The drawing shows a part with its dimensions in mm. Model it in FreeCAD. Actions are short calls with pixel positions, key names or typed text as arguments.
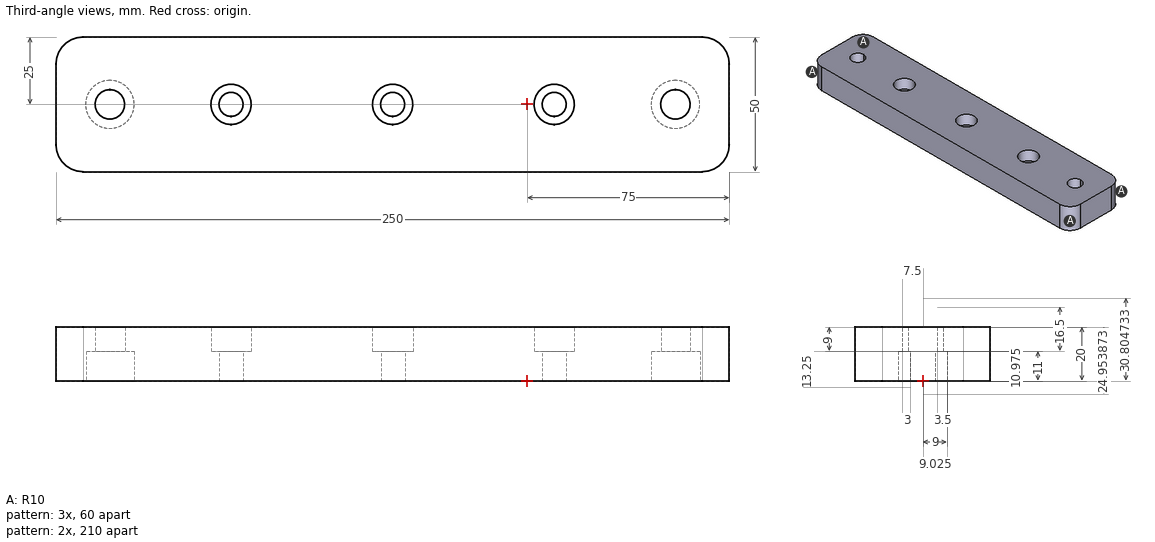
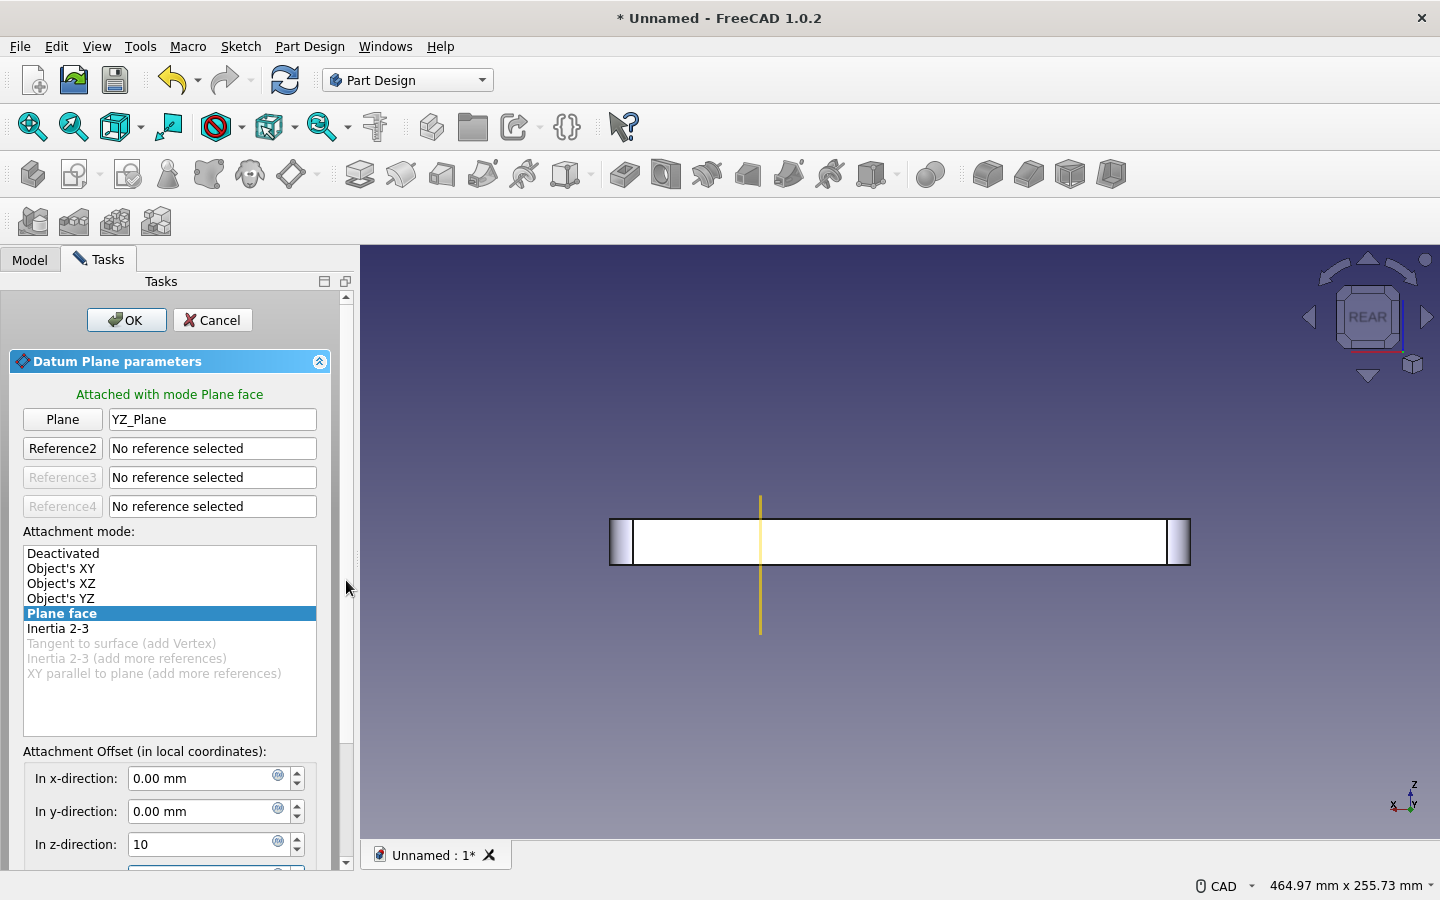
click(127, 320)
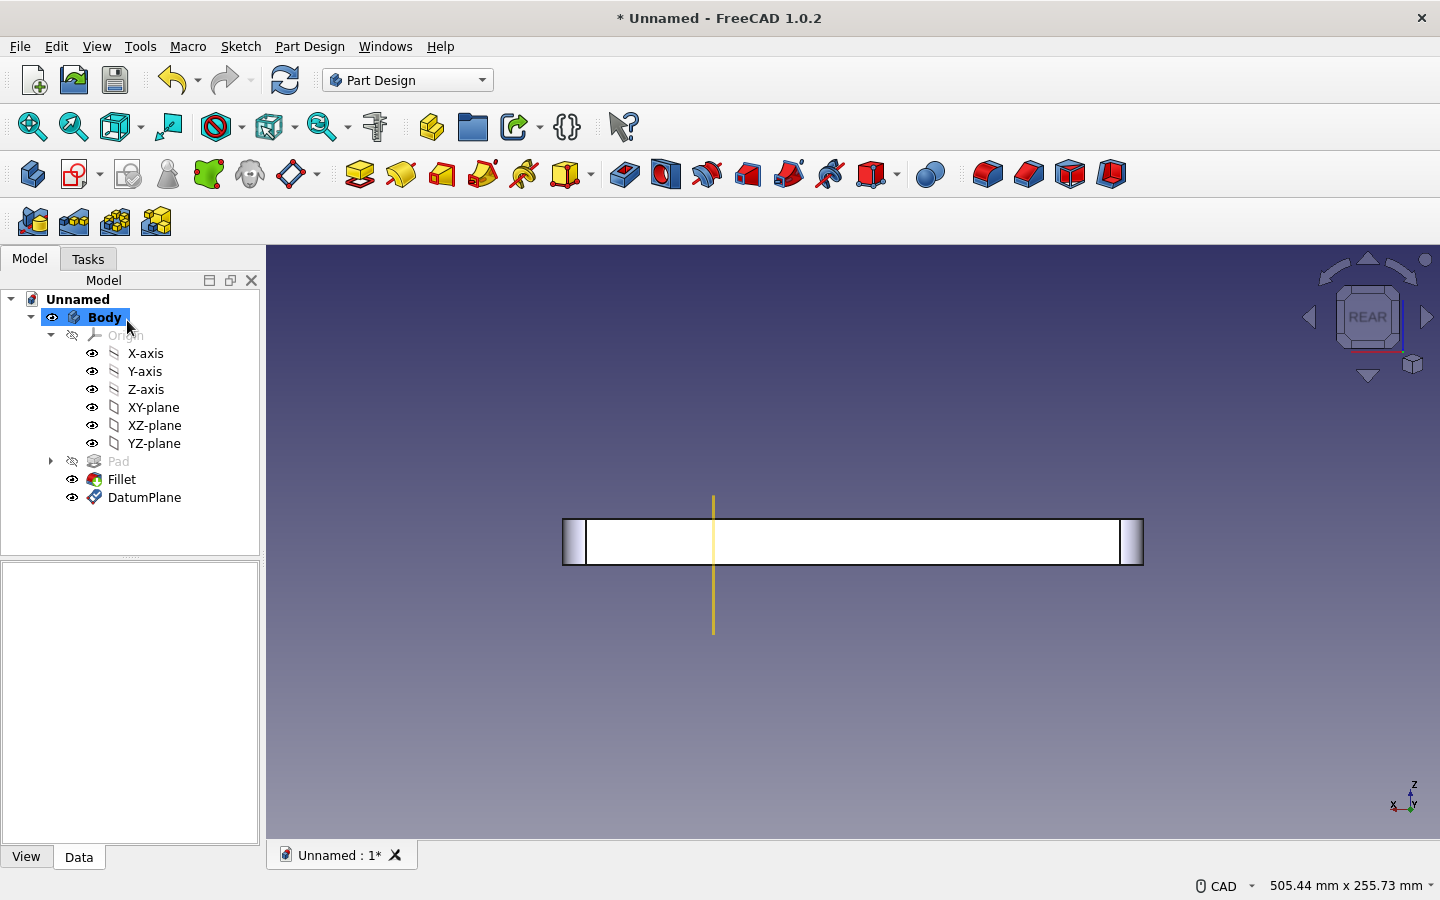
click(117, 497)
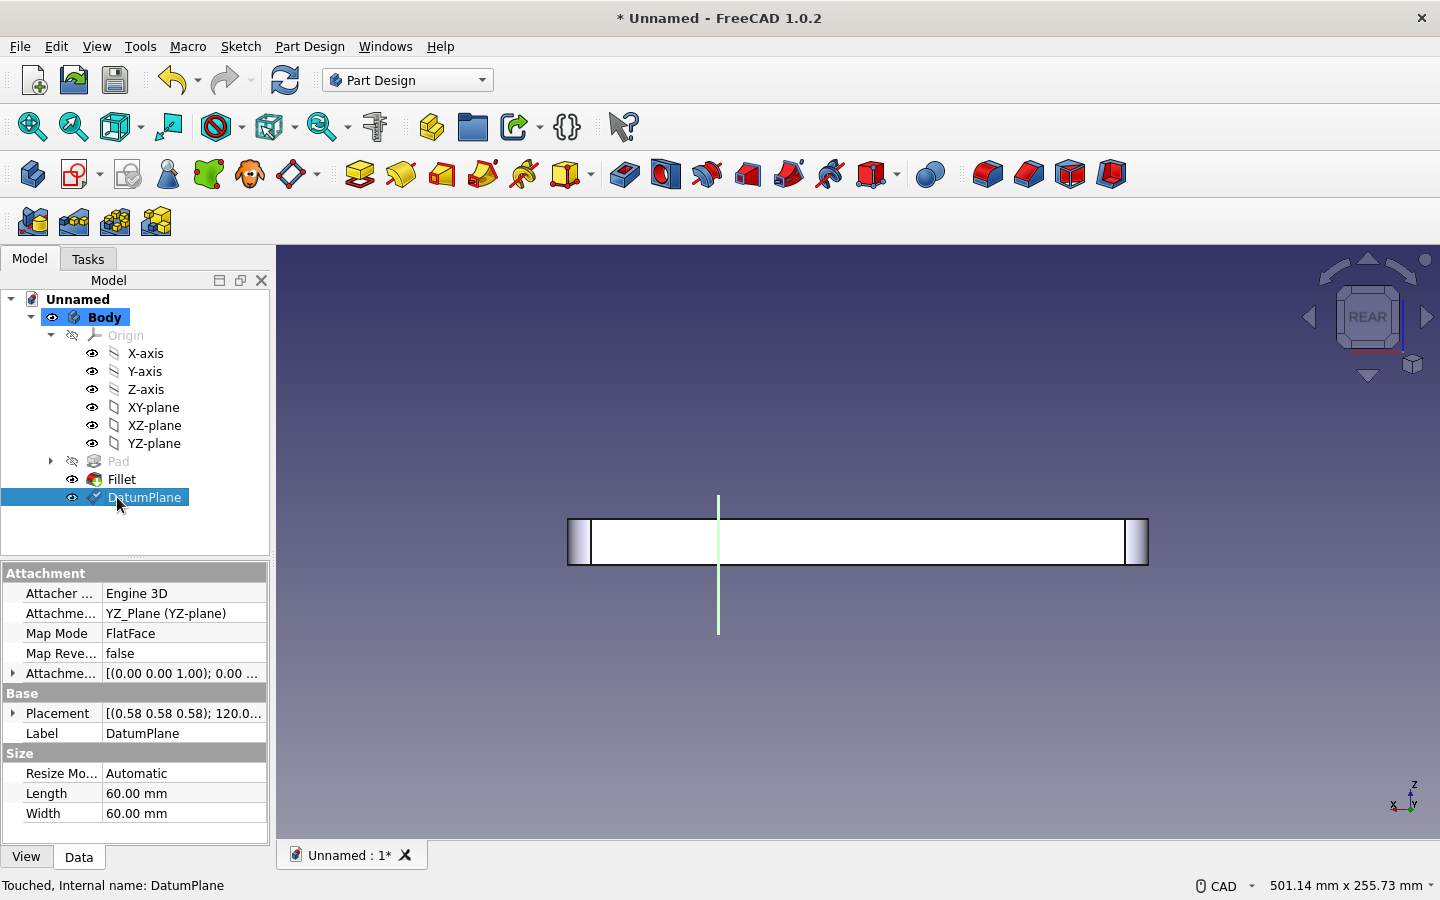
click(74, 174)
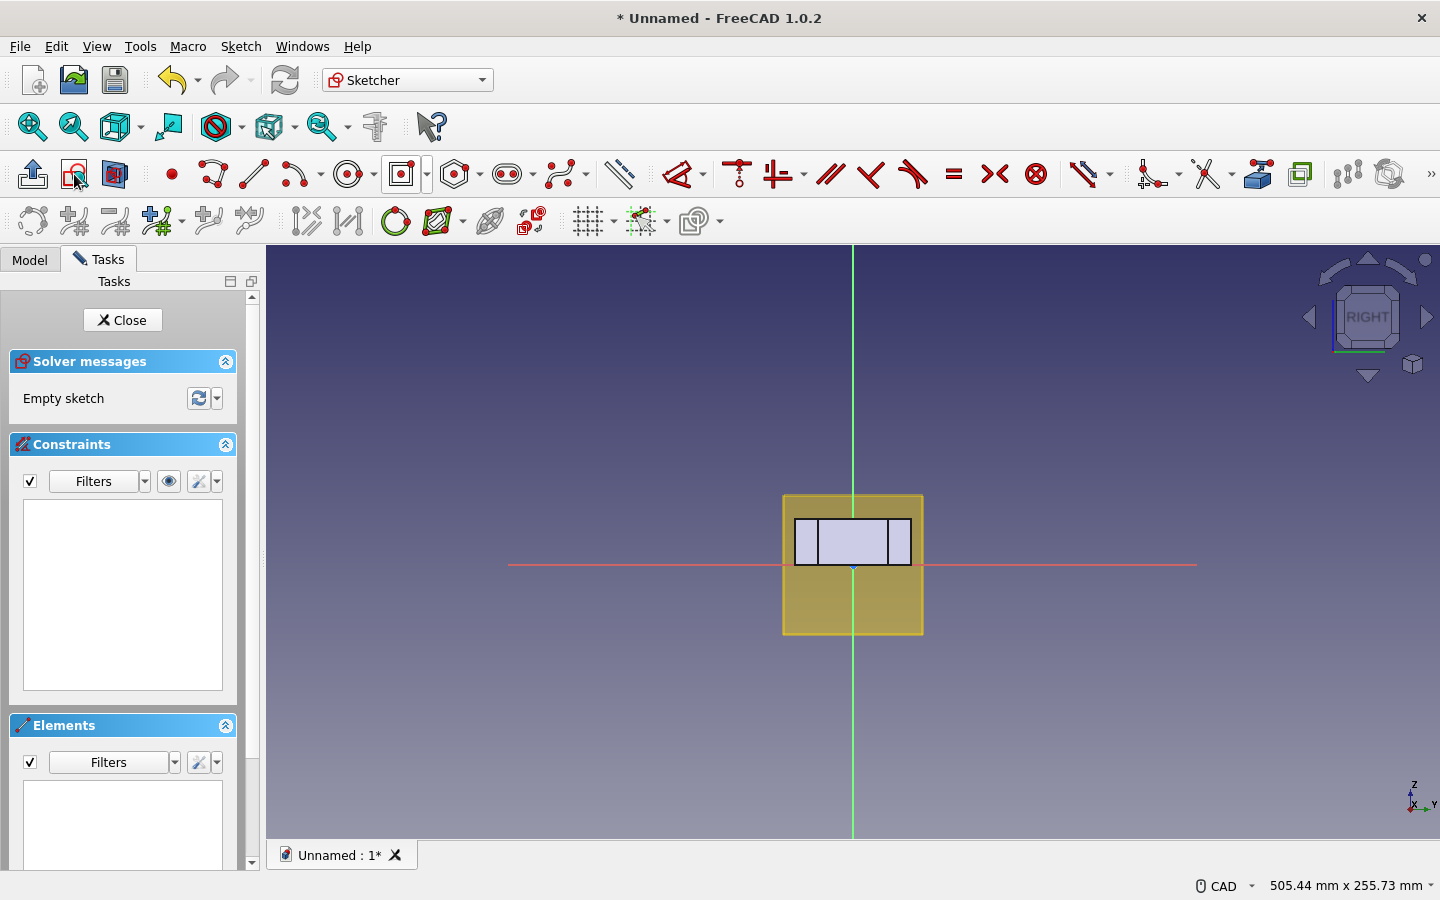
key(q)
key(s)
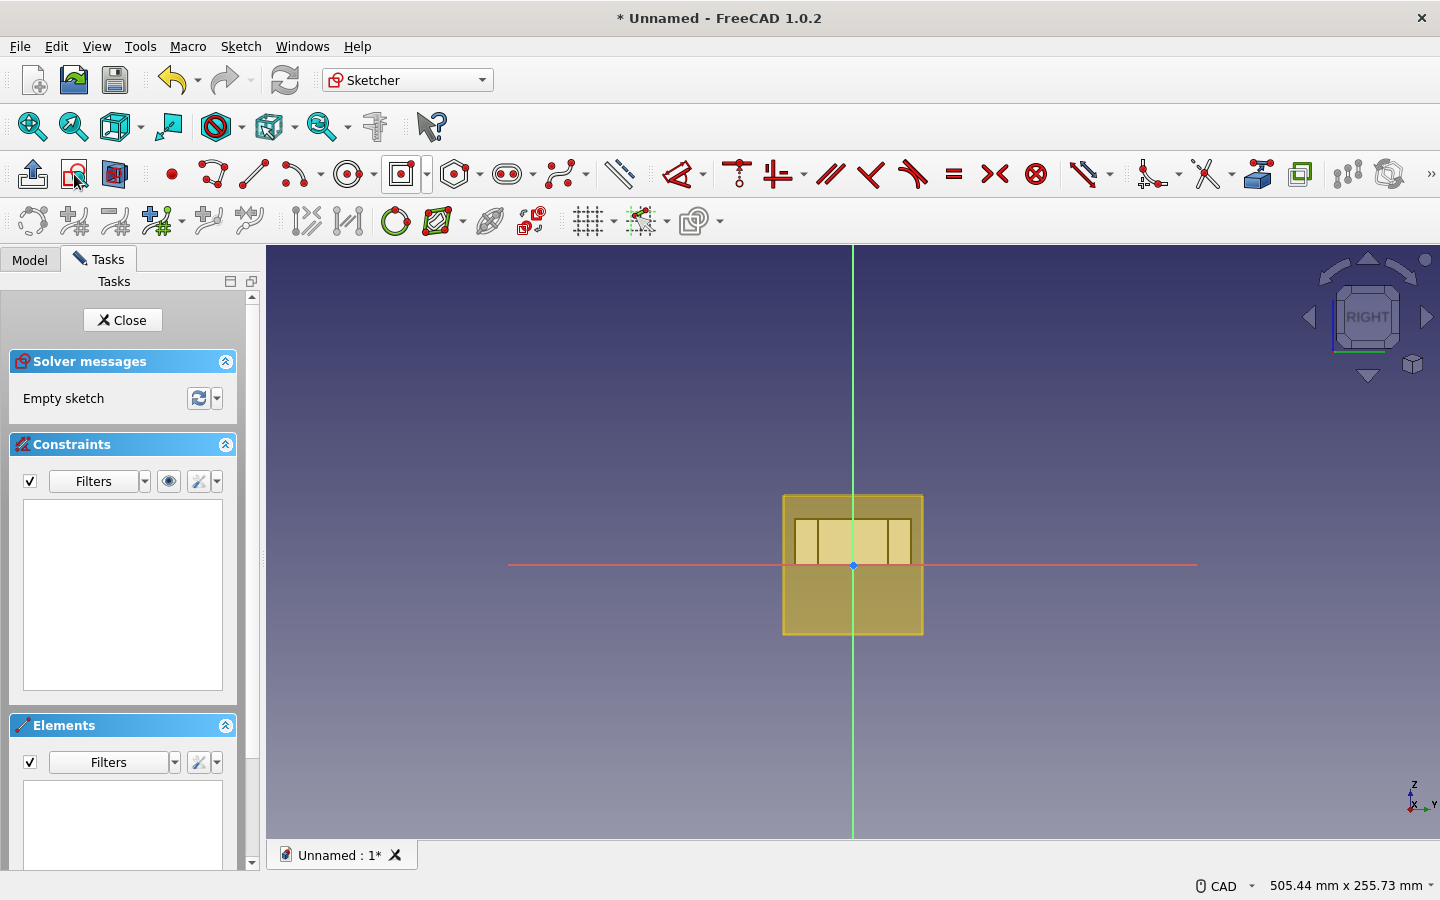
scroll(856, 549, up, 9)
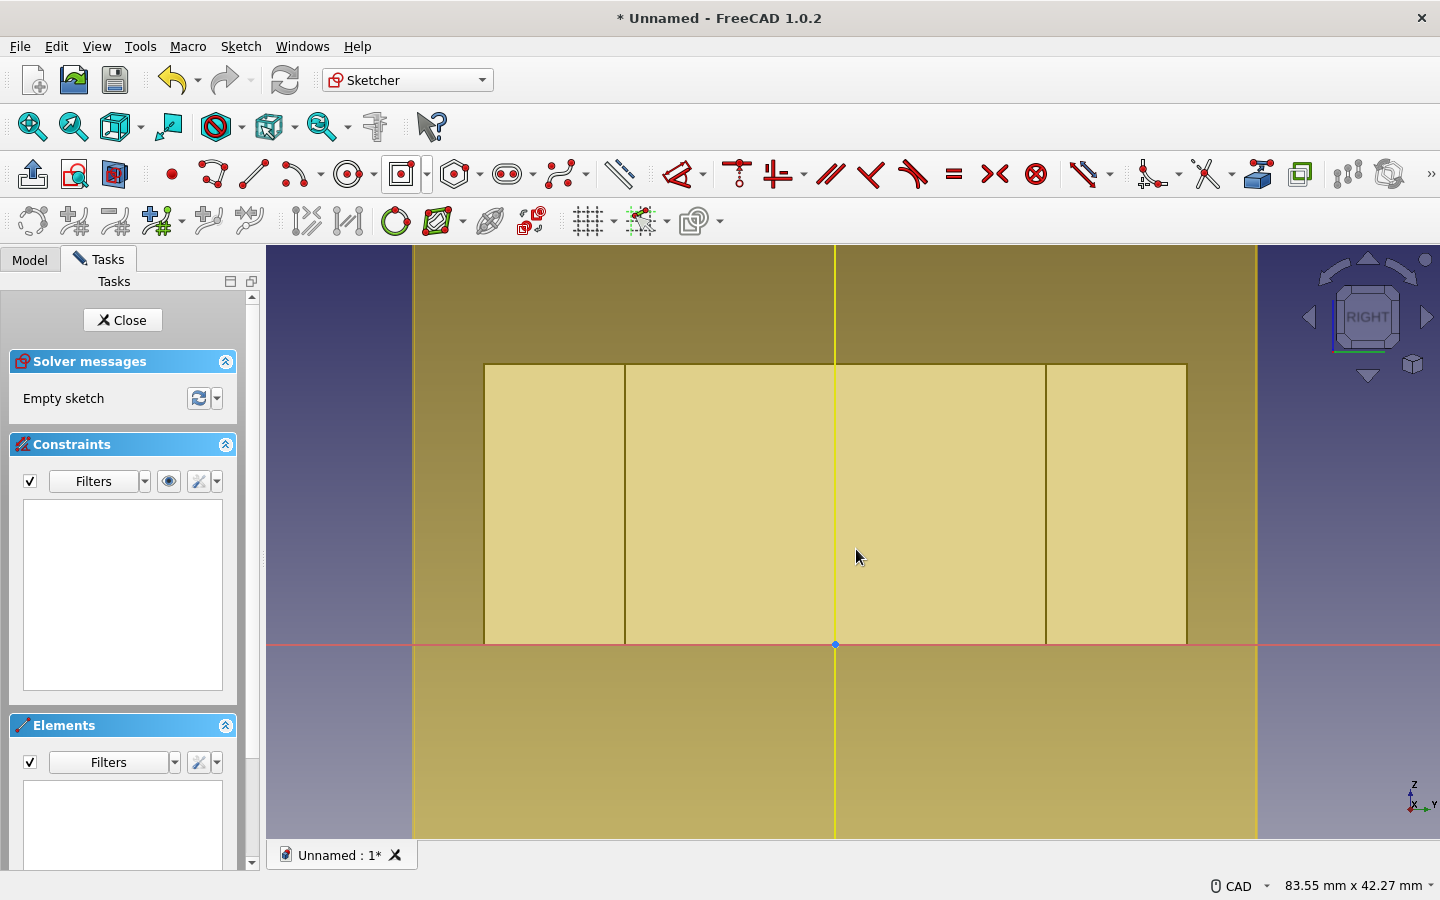
key(g)
key(m)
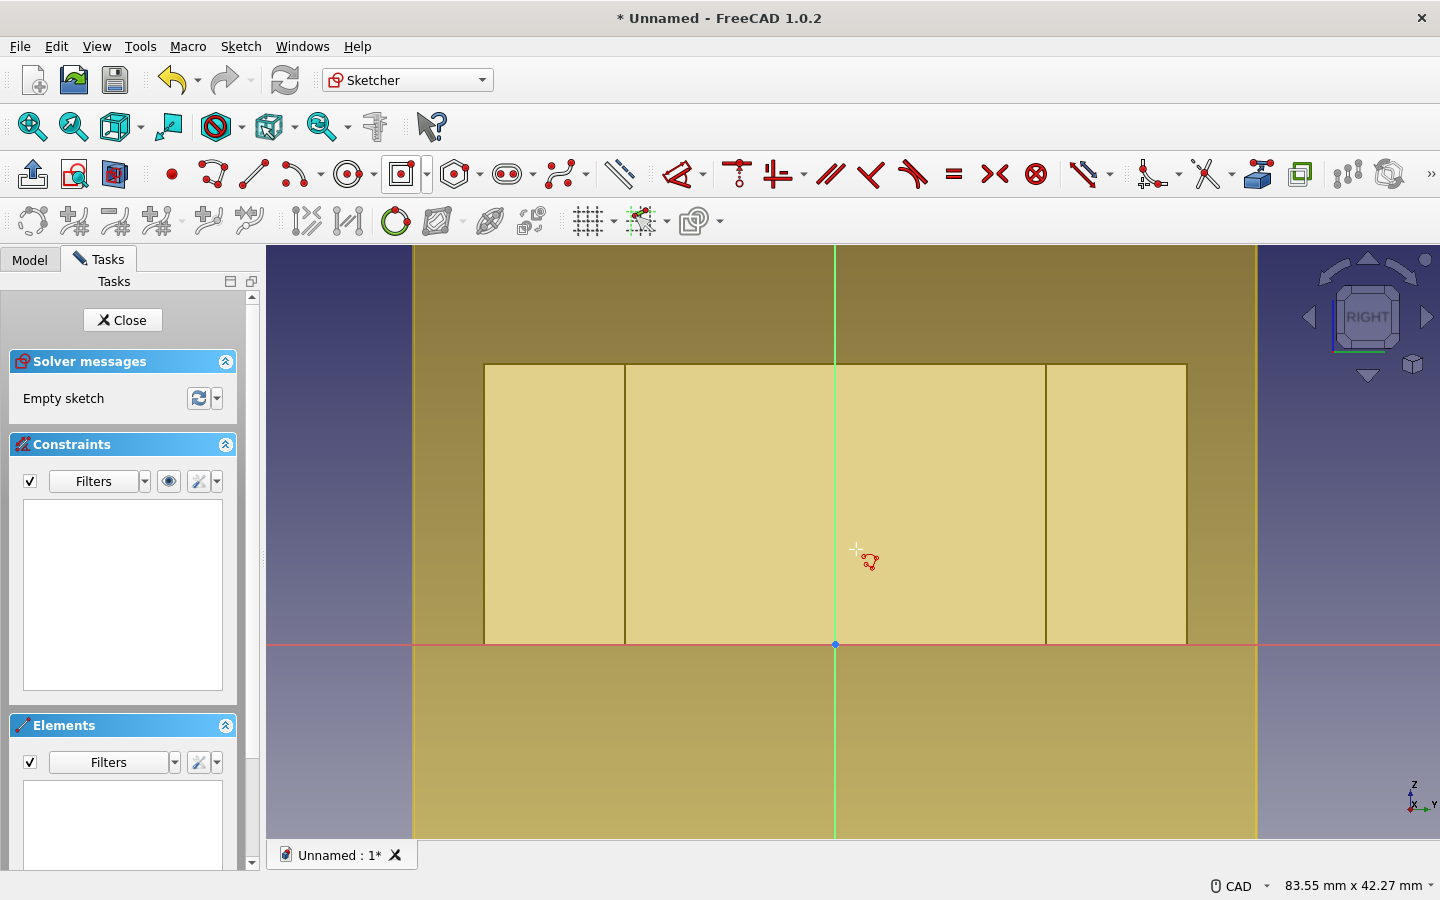
click(835, 714)
click(826, 364)
click(730, 364)
click(730, 490)
click(772, 490)
click(772, 676)
click(835, 715)
key(Escape)
key(Escape)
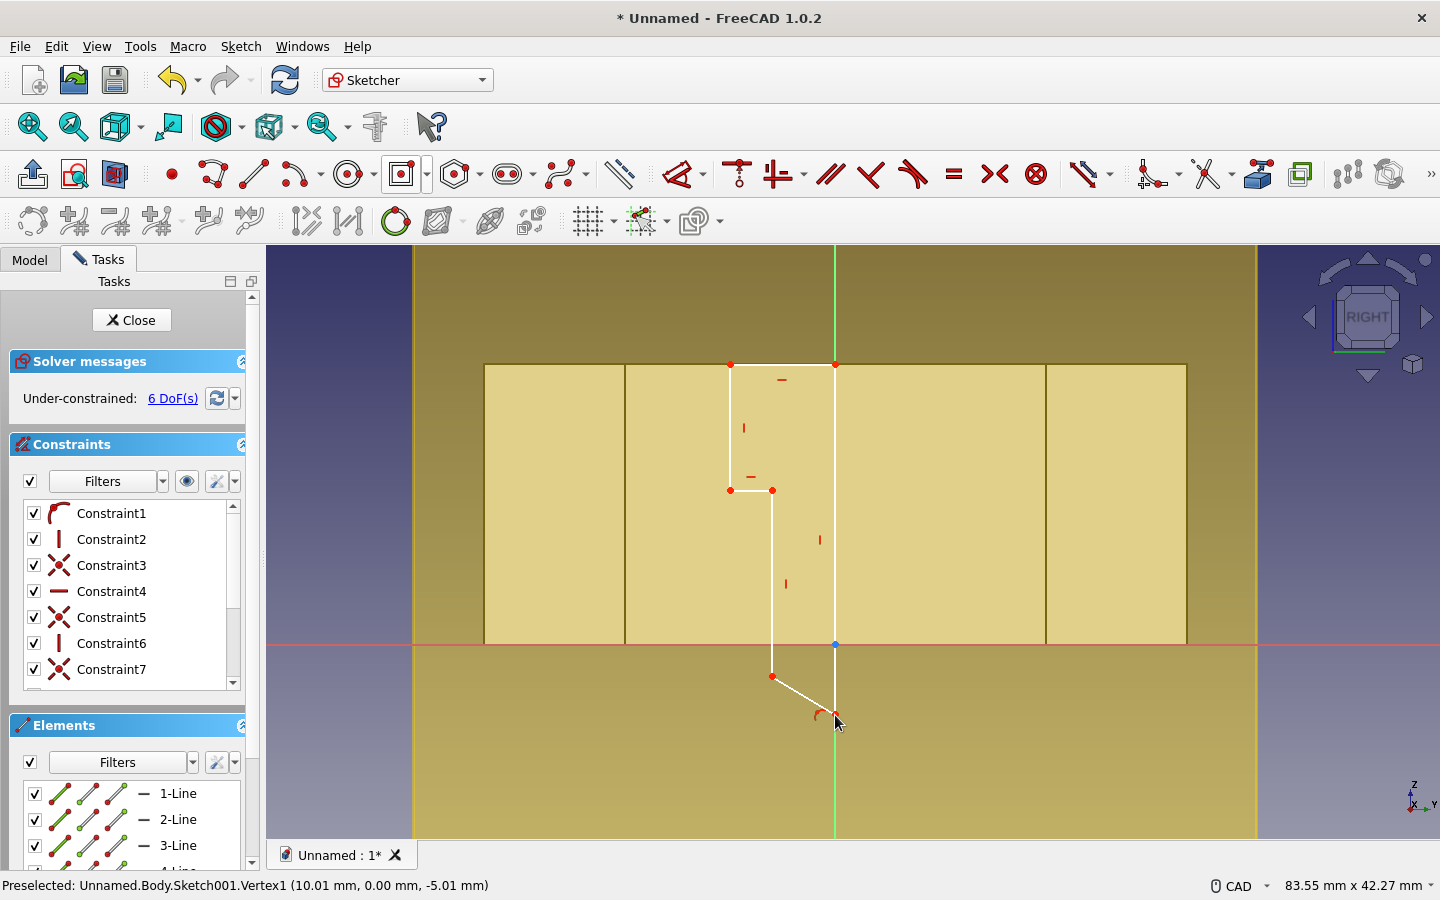
click(730, 403)